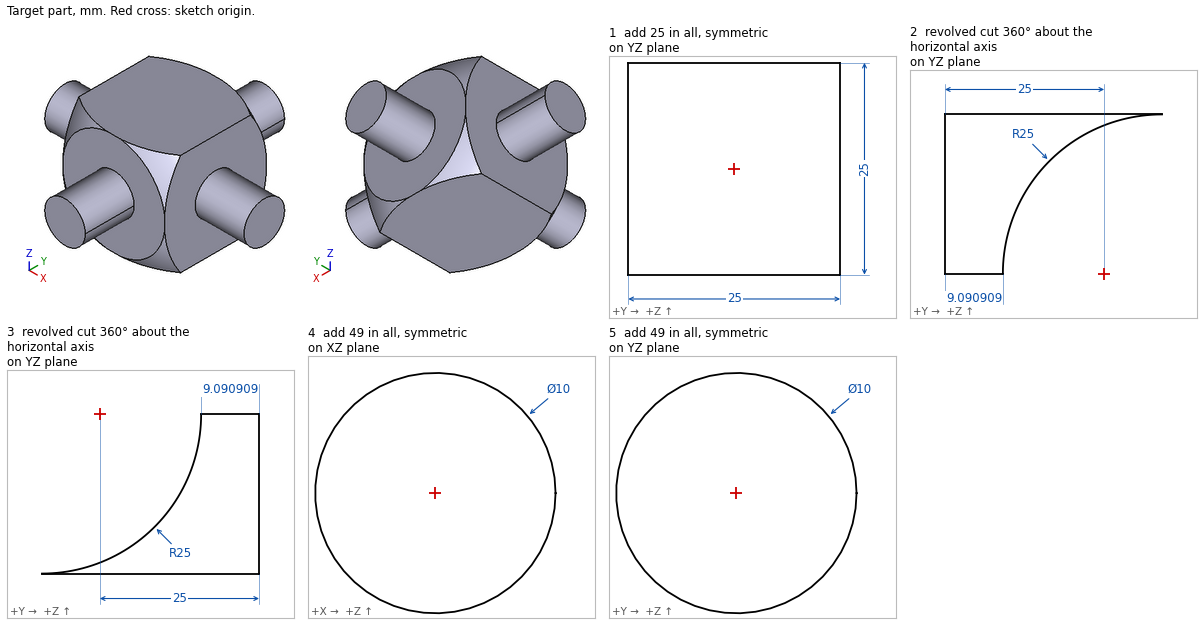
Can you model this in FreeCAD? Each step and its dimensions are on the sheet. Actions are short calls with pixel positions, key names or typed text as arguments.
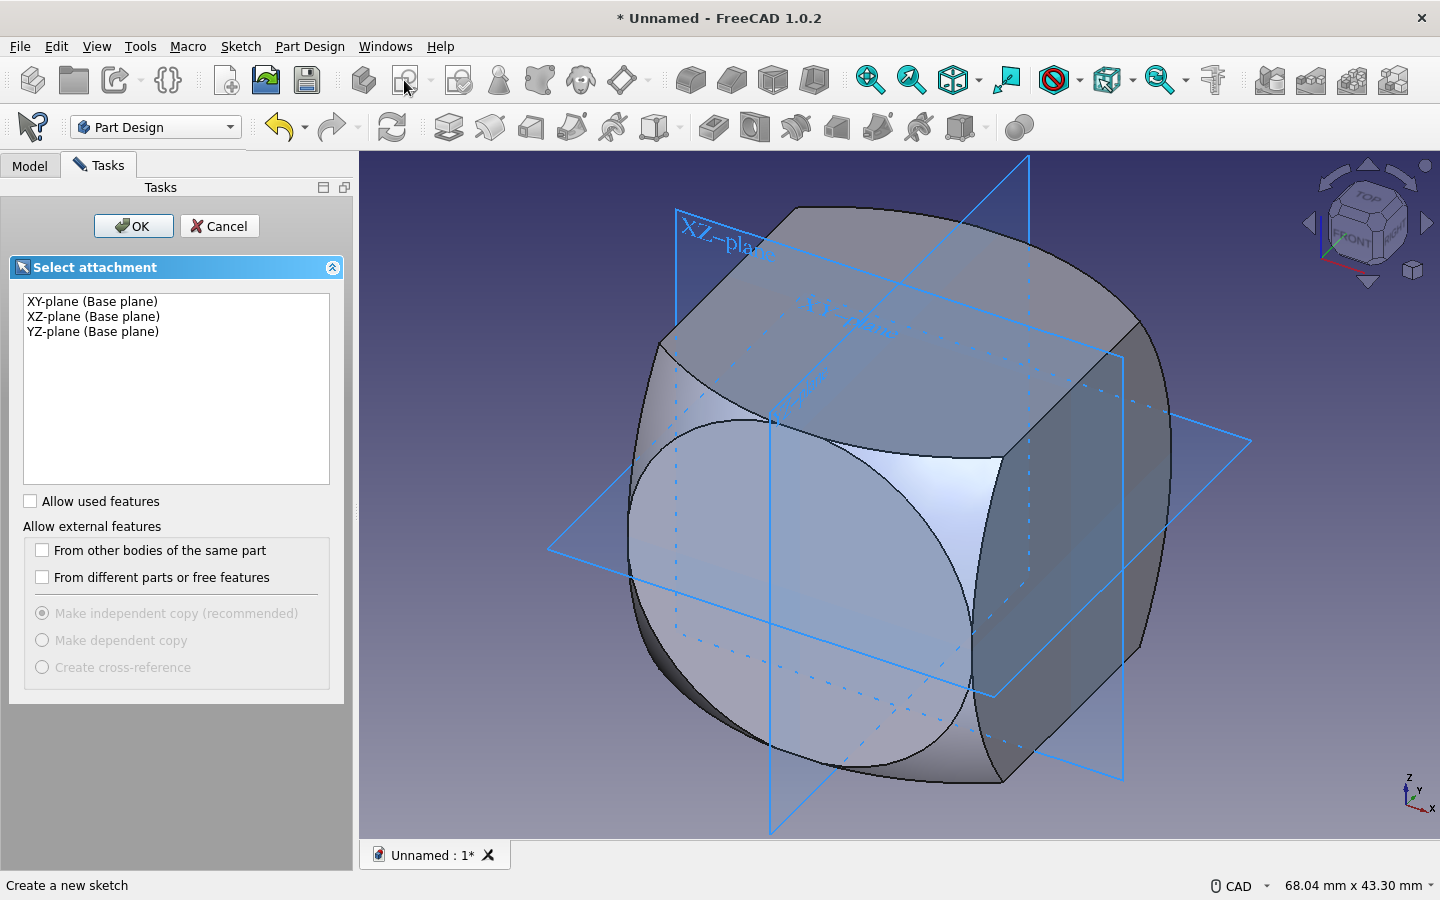
click(84, 316)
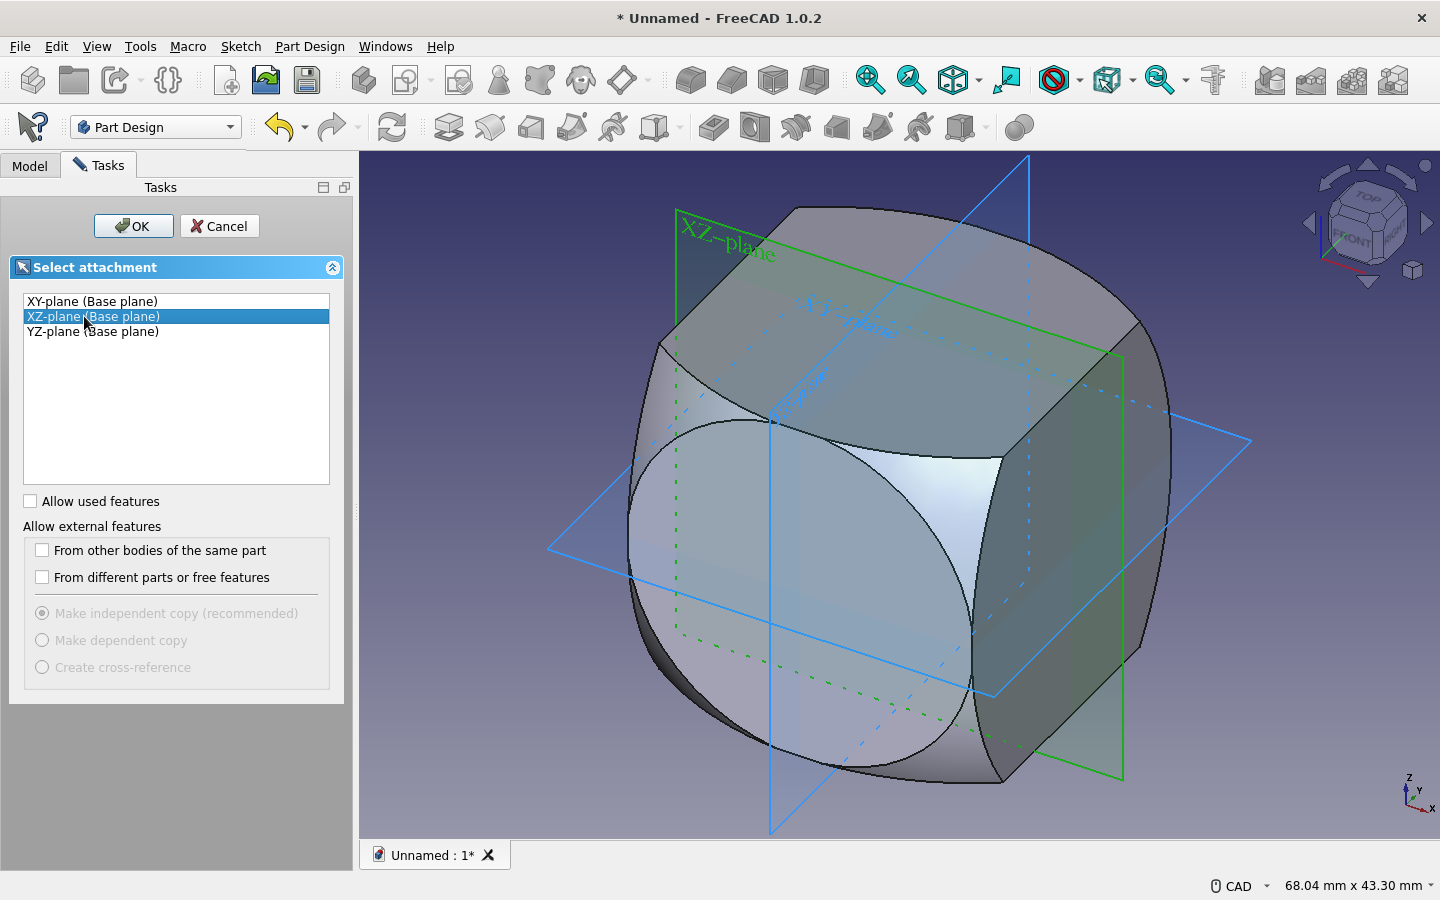
click(134, 226)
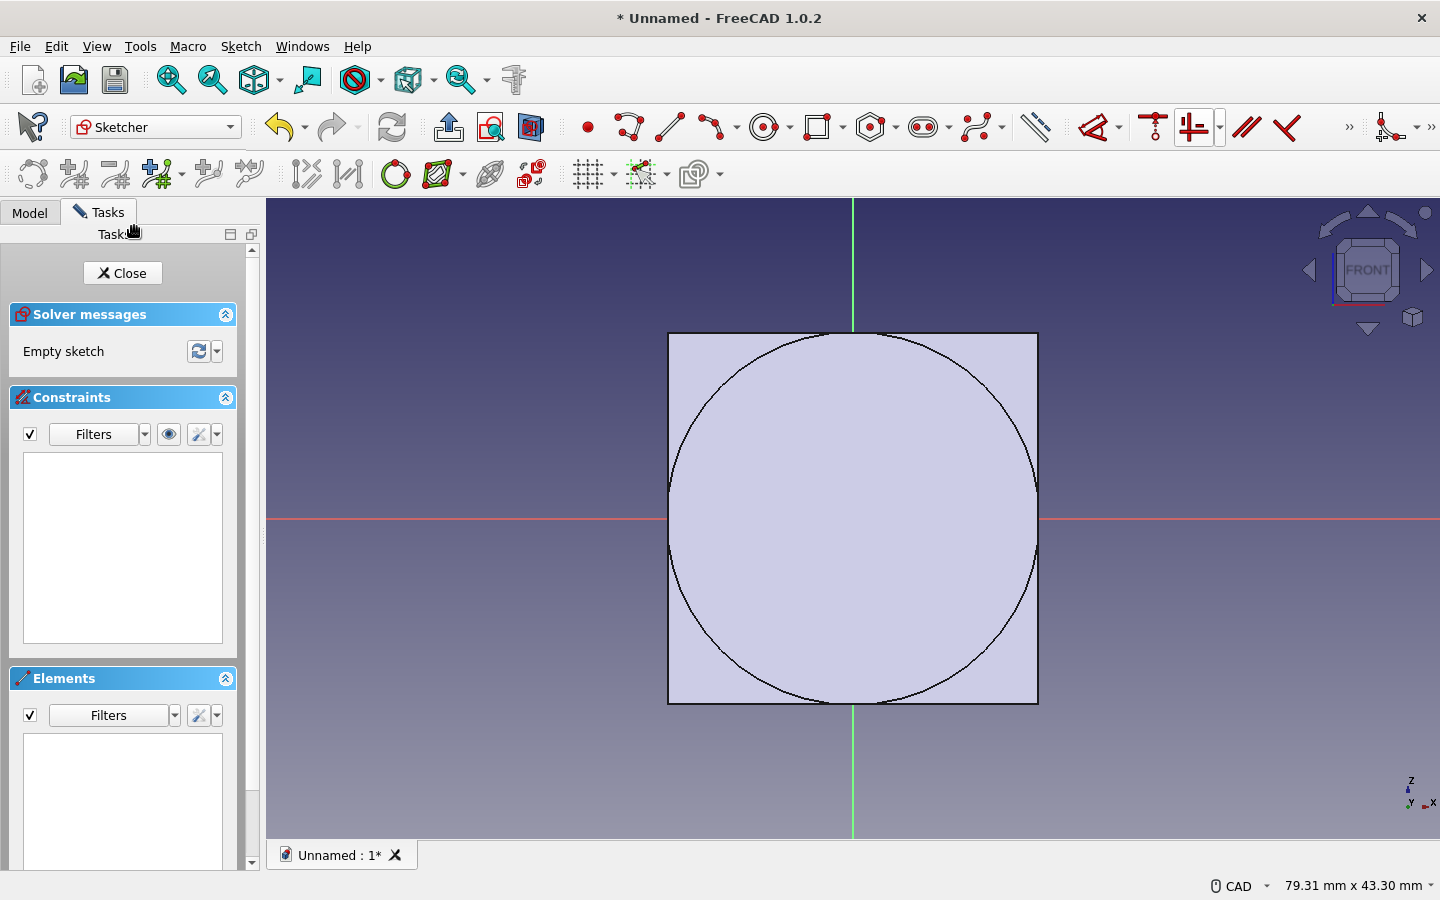
key(q)
key(s)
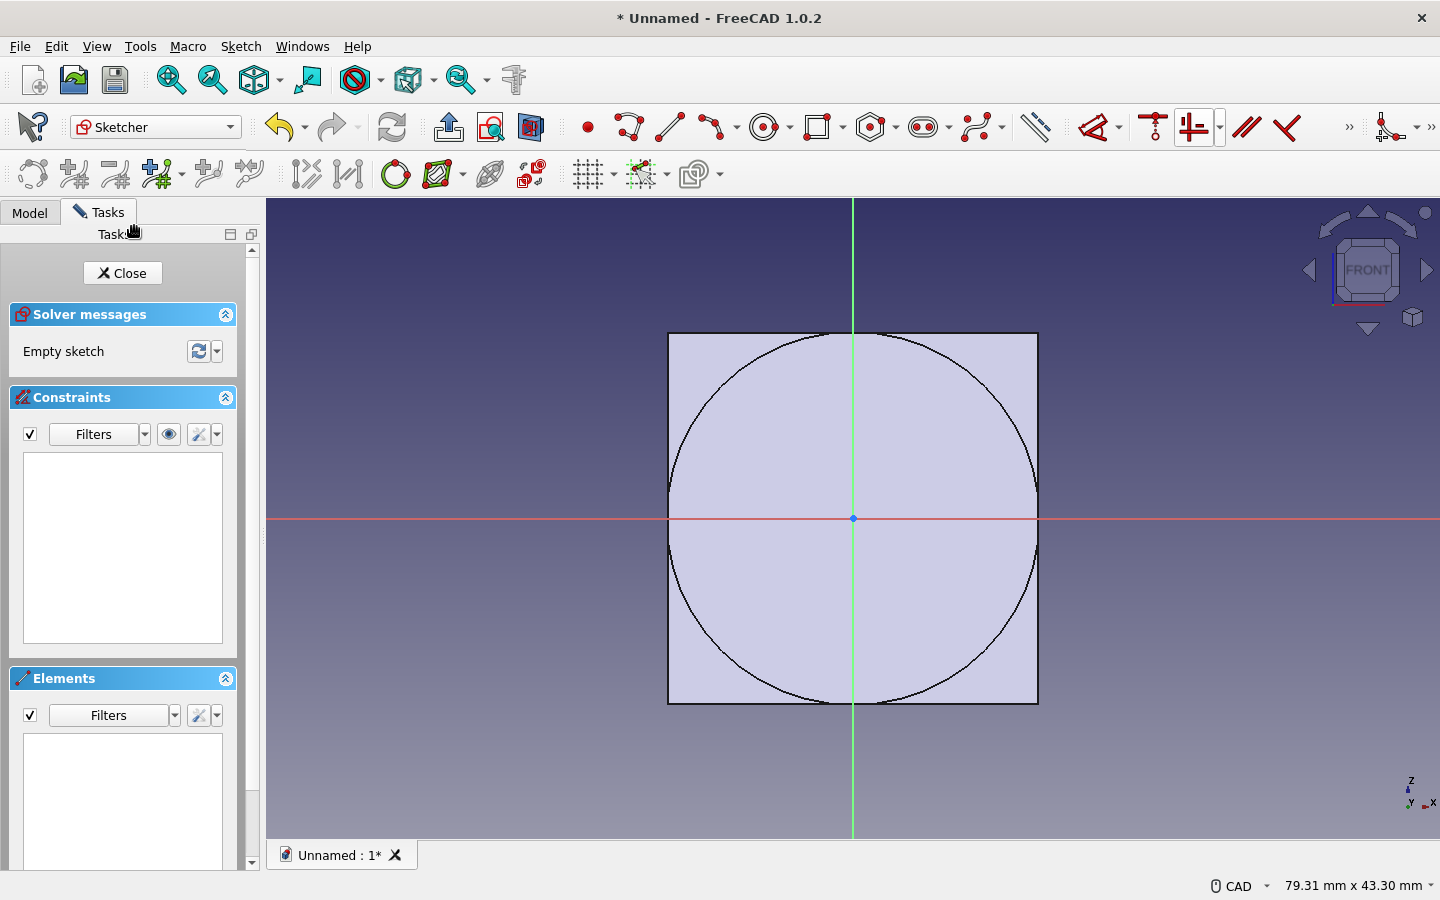
scroll(893, 518, up, 5)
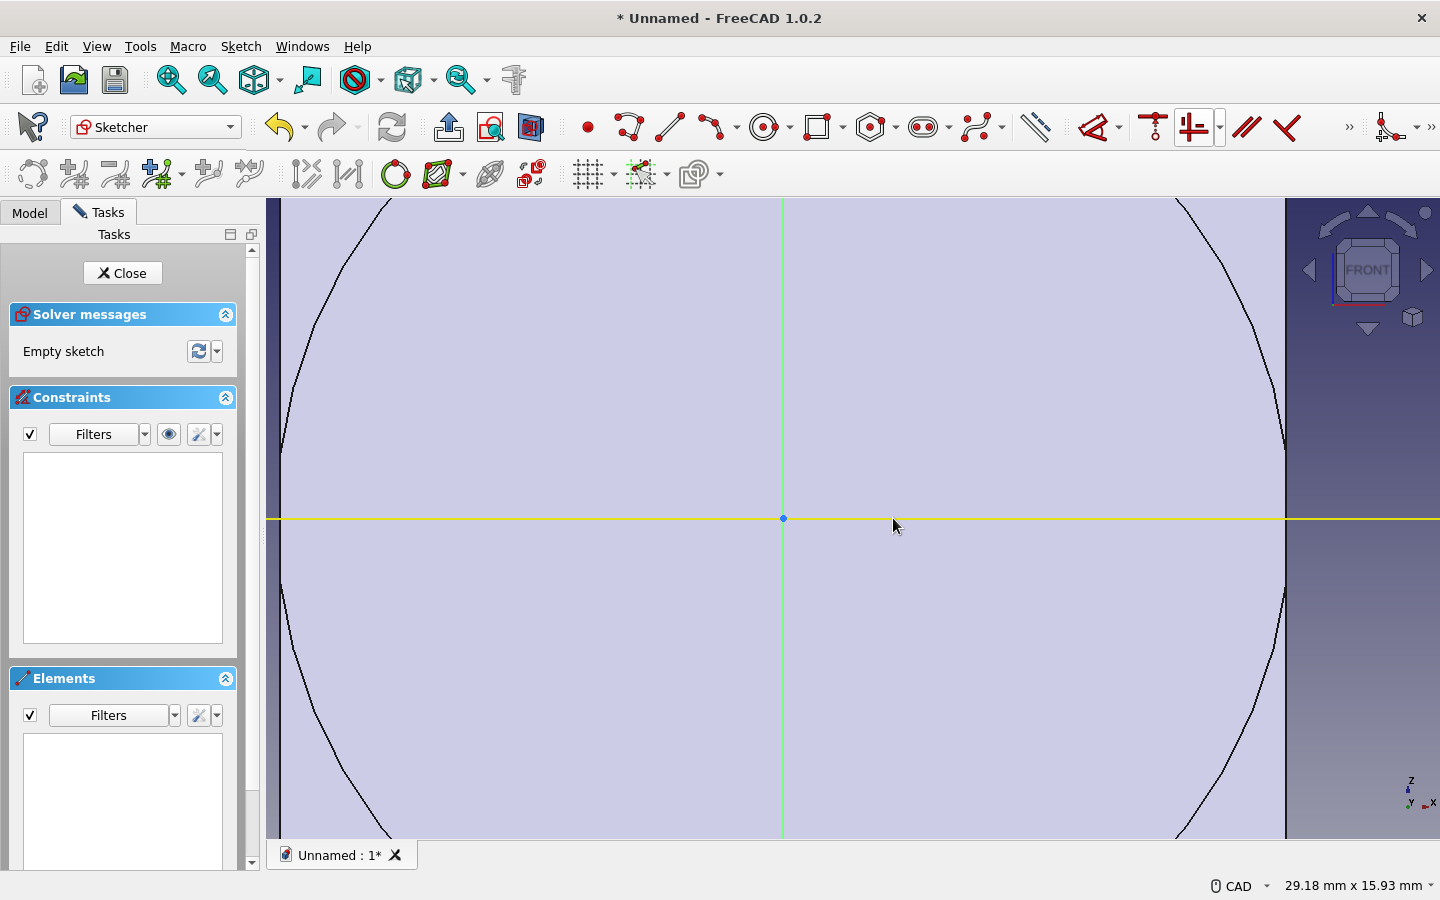
key(g)
key(c)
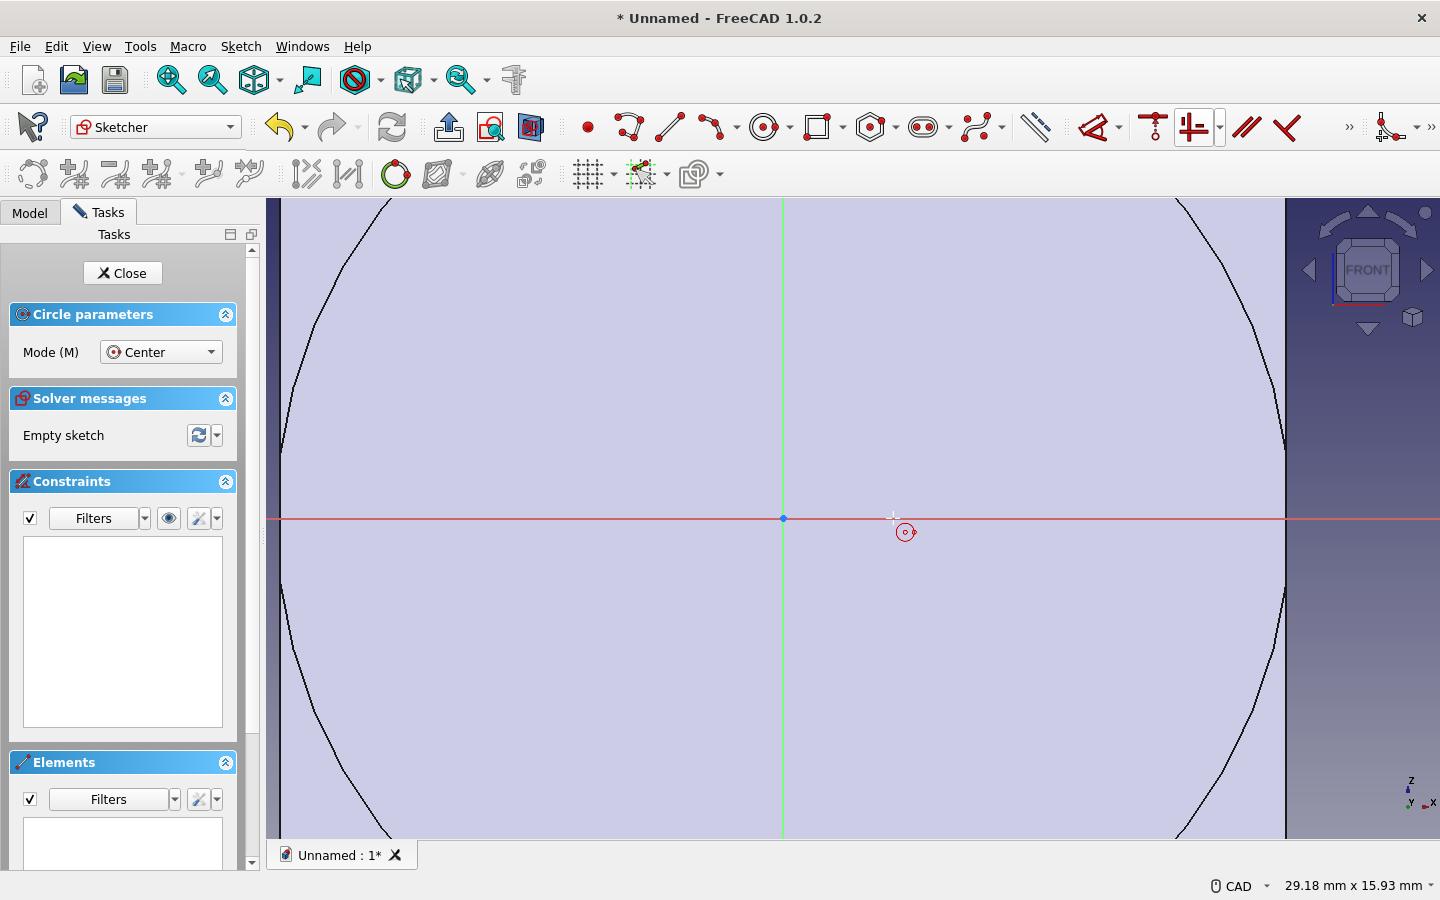
click(783, 518)
click(926, 376)
key(Escape)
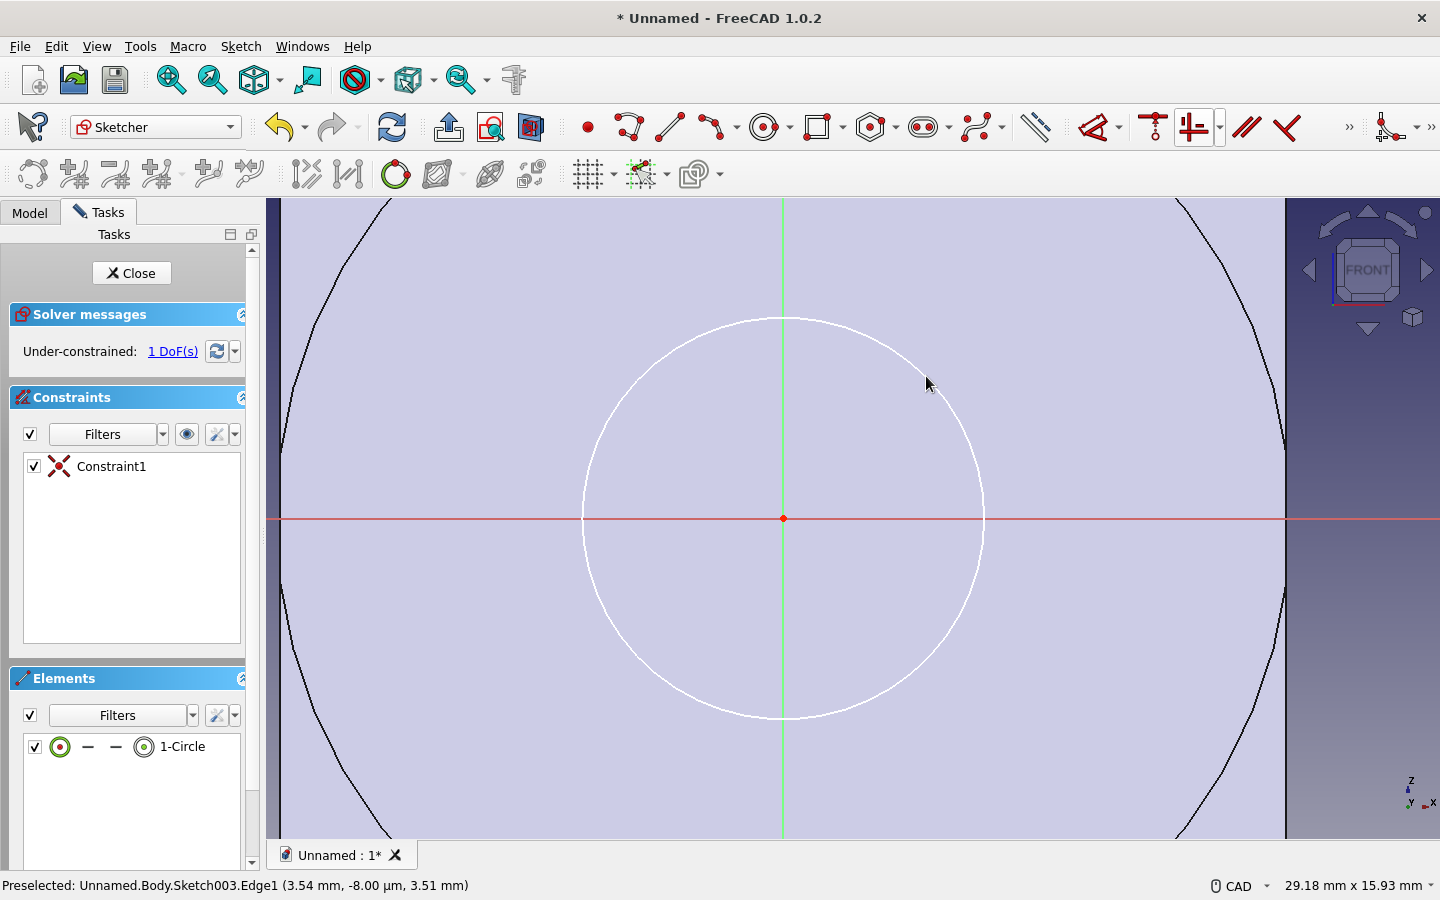
click(1092, 128)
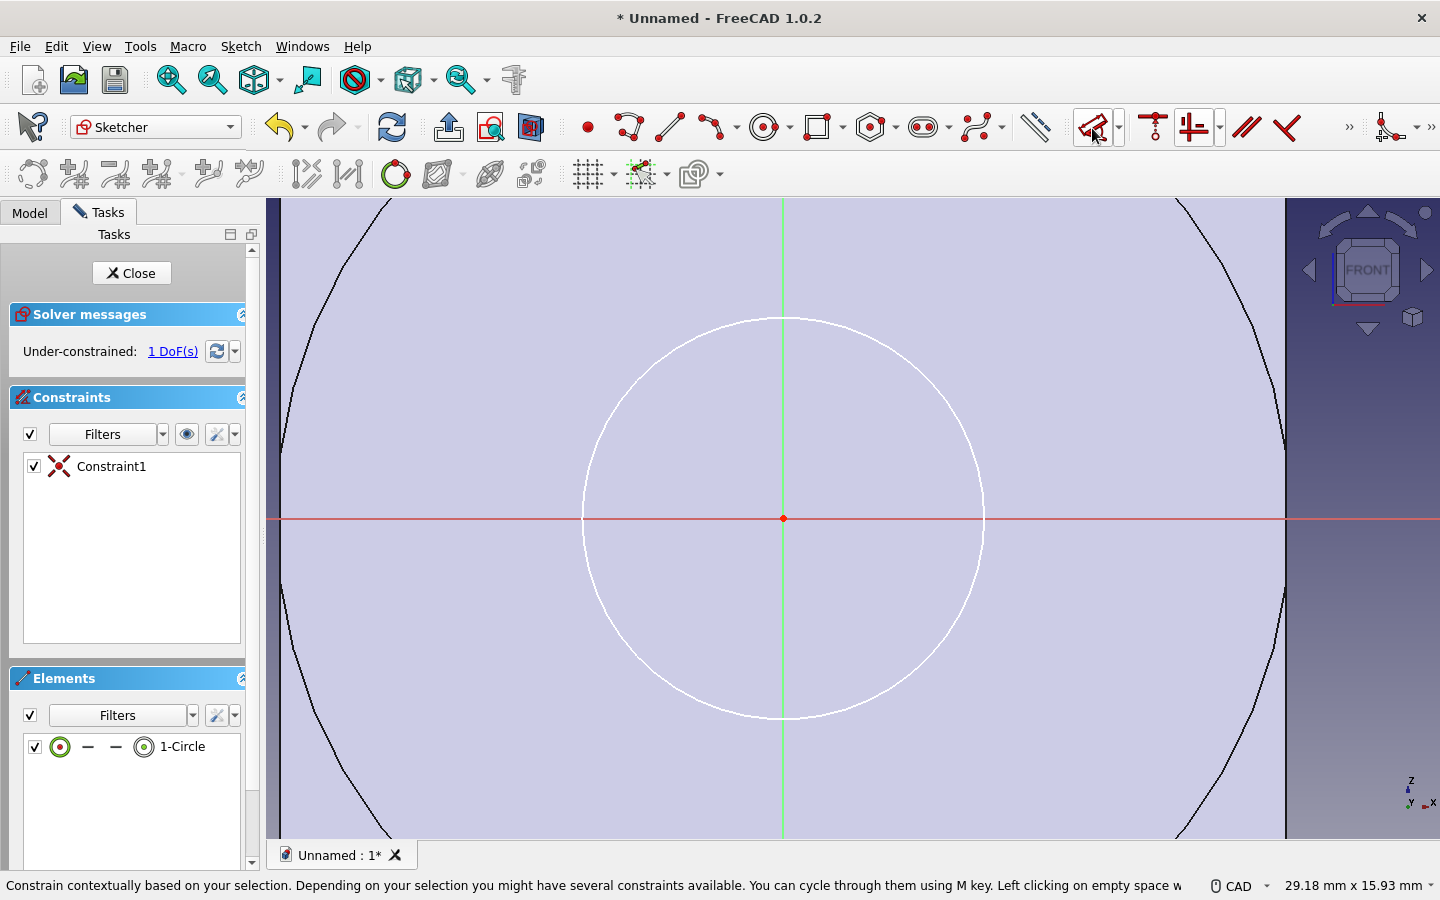
click(925, 376)
click(948, 353)